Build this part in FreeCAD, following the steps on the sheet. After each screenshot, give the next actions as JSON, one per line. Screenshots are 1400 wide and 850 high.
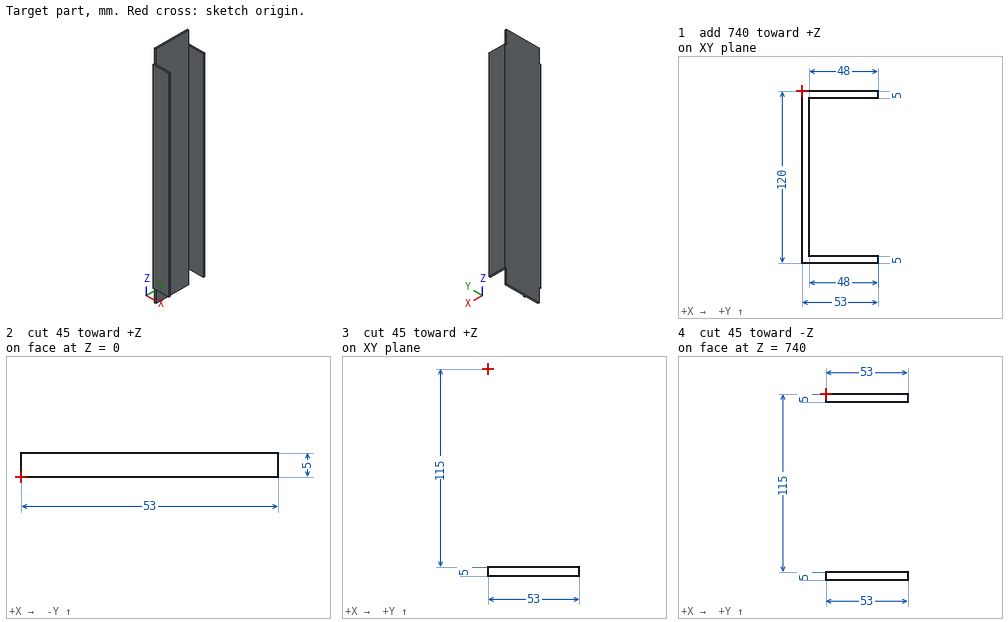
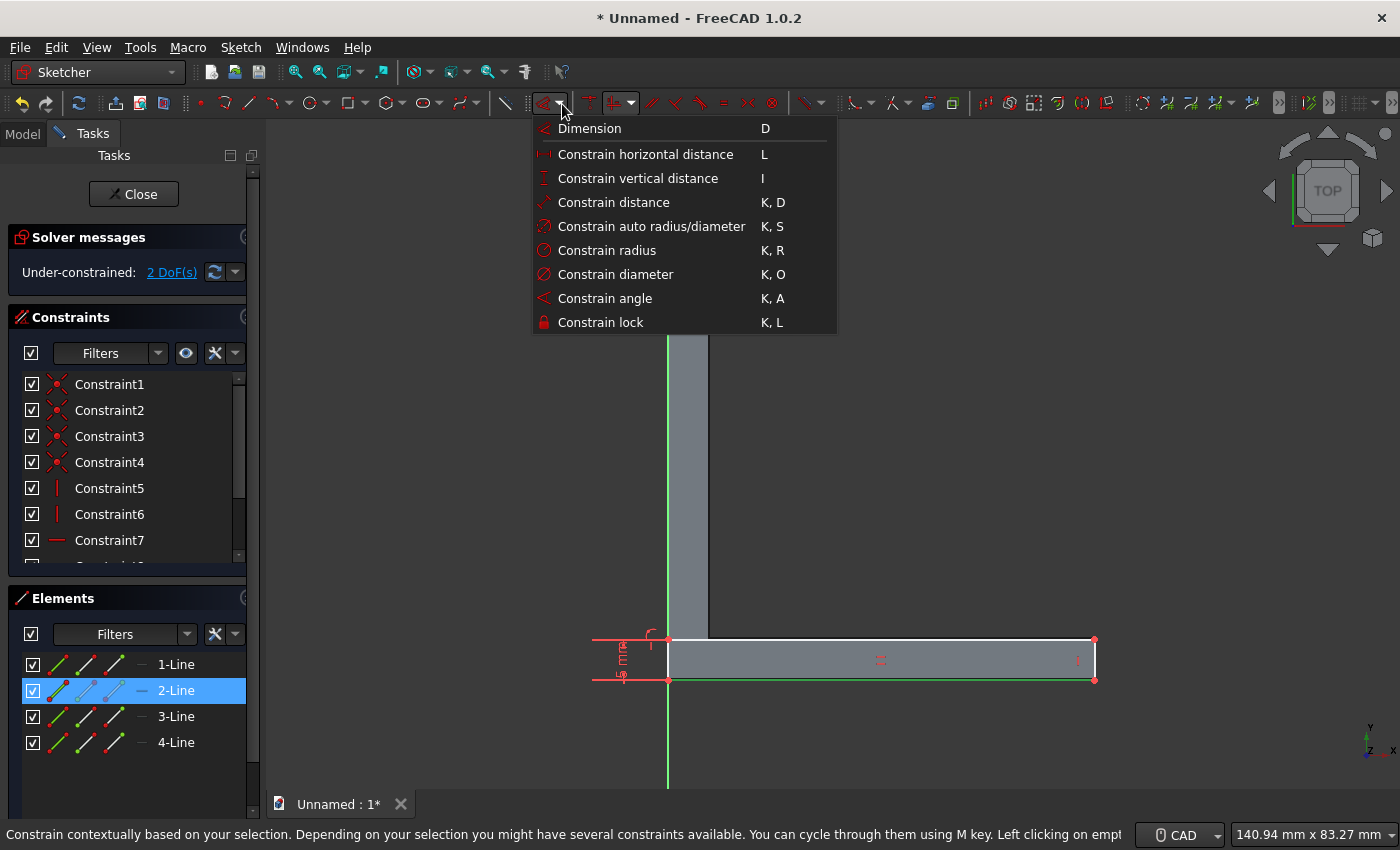
{"action": "left_click", "coordinate": [685, 154]}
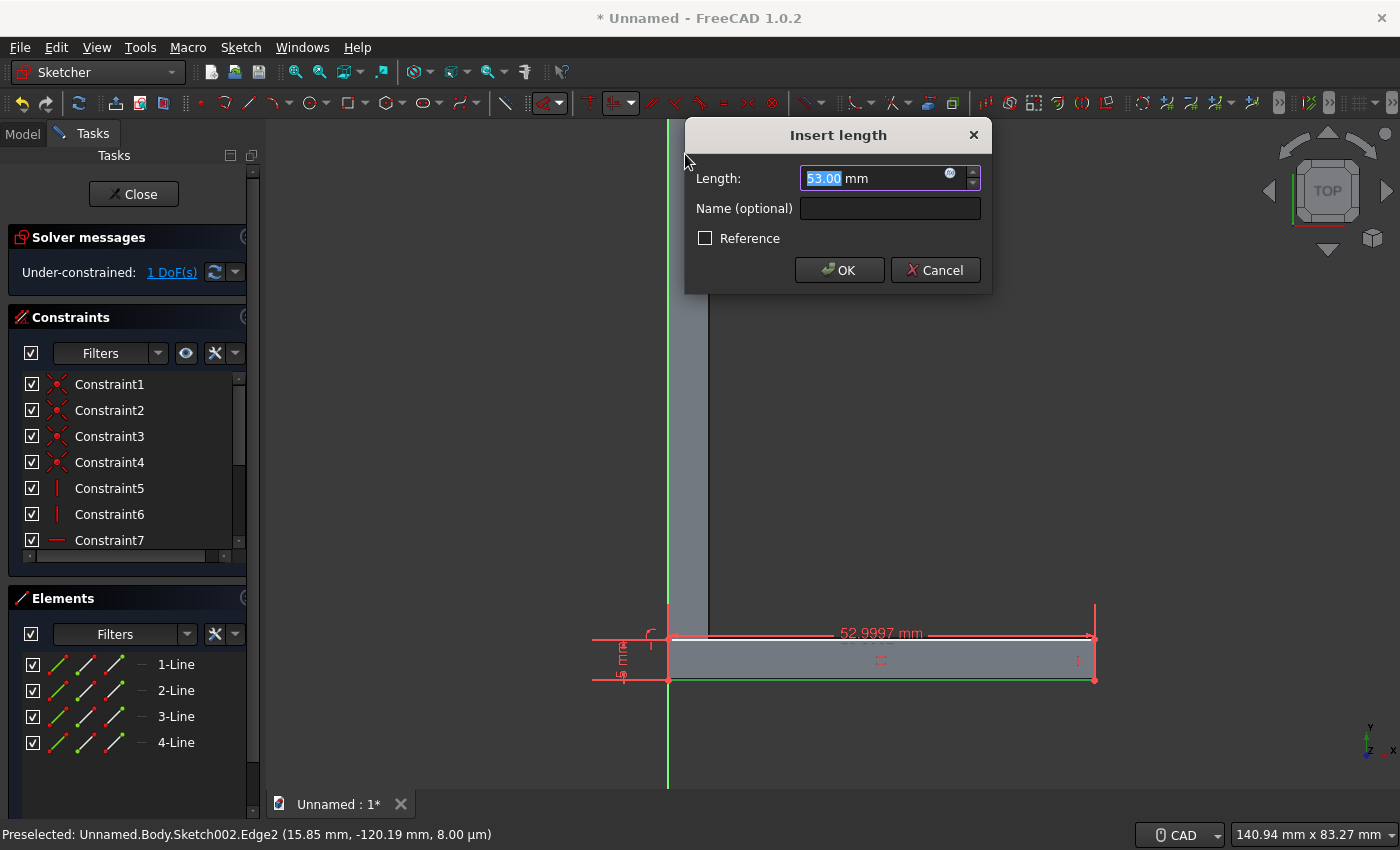
{"action": "type", "text": "53"}
{"action": "key", "text": "Return"}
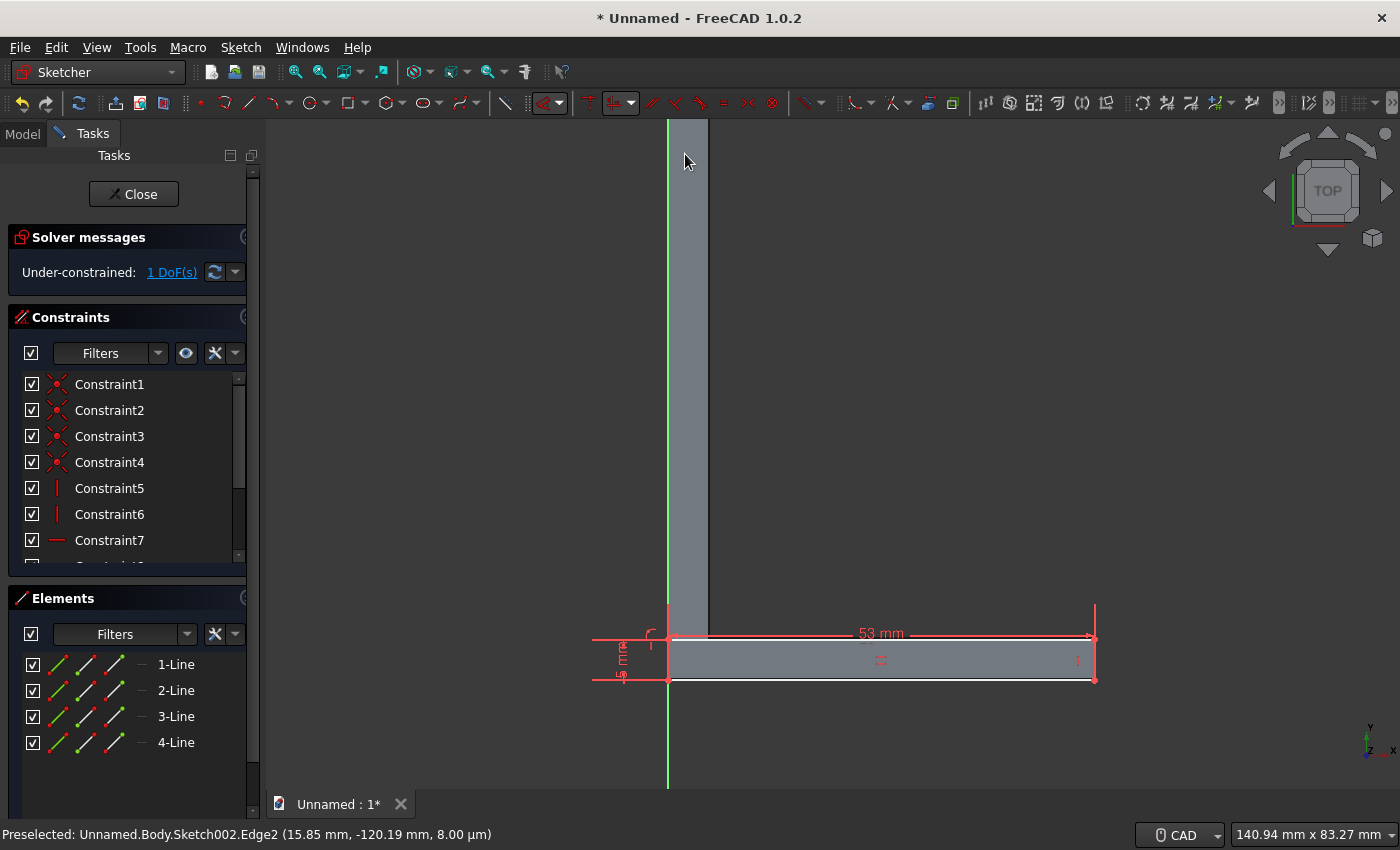
{"action": "left_click", "coordinate": [668, 640]}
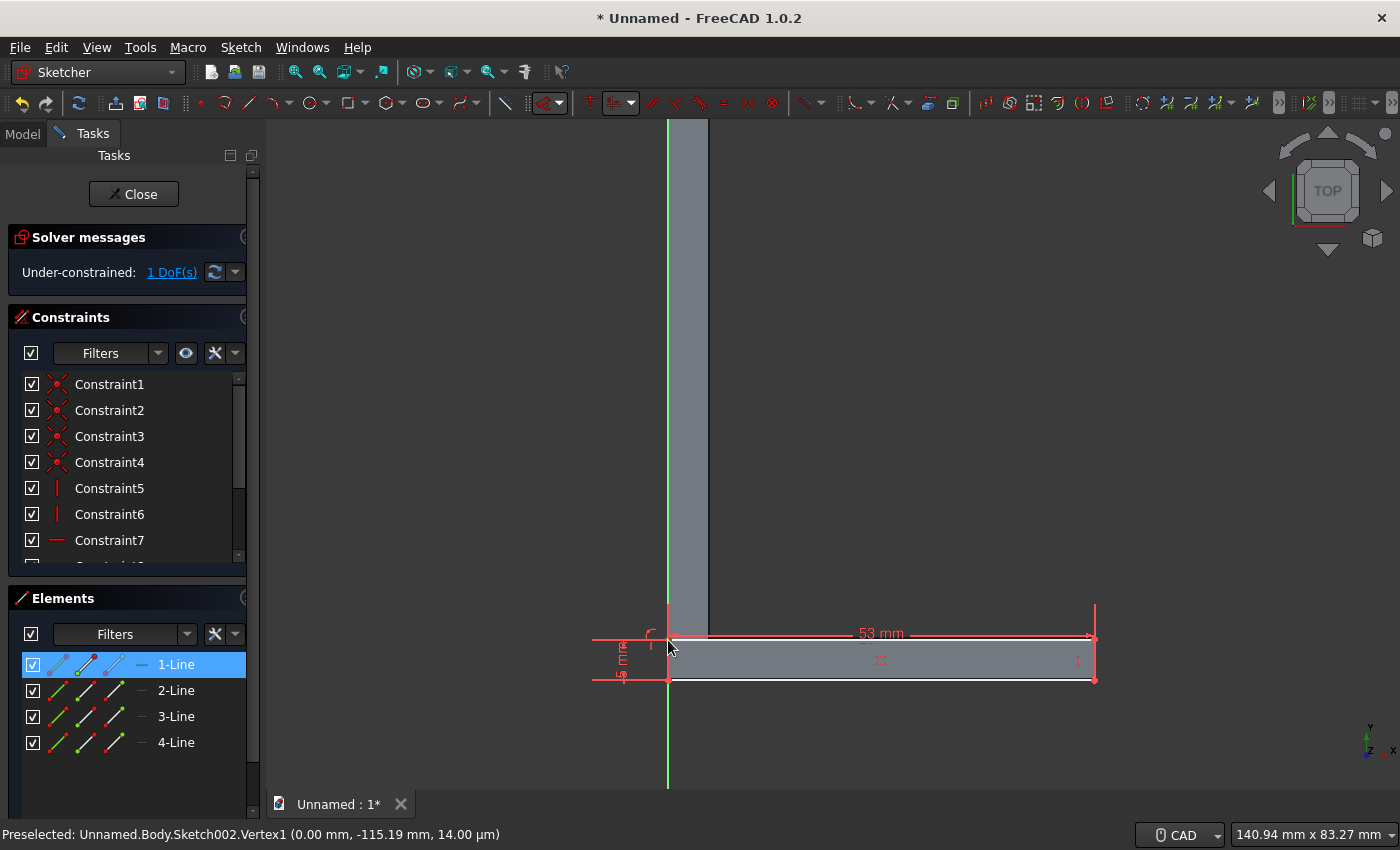
{"action": "key", "text": "i"}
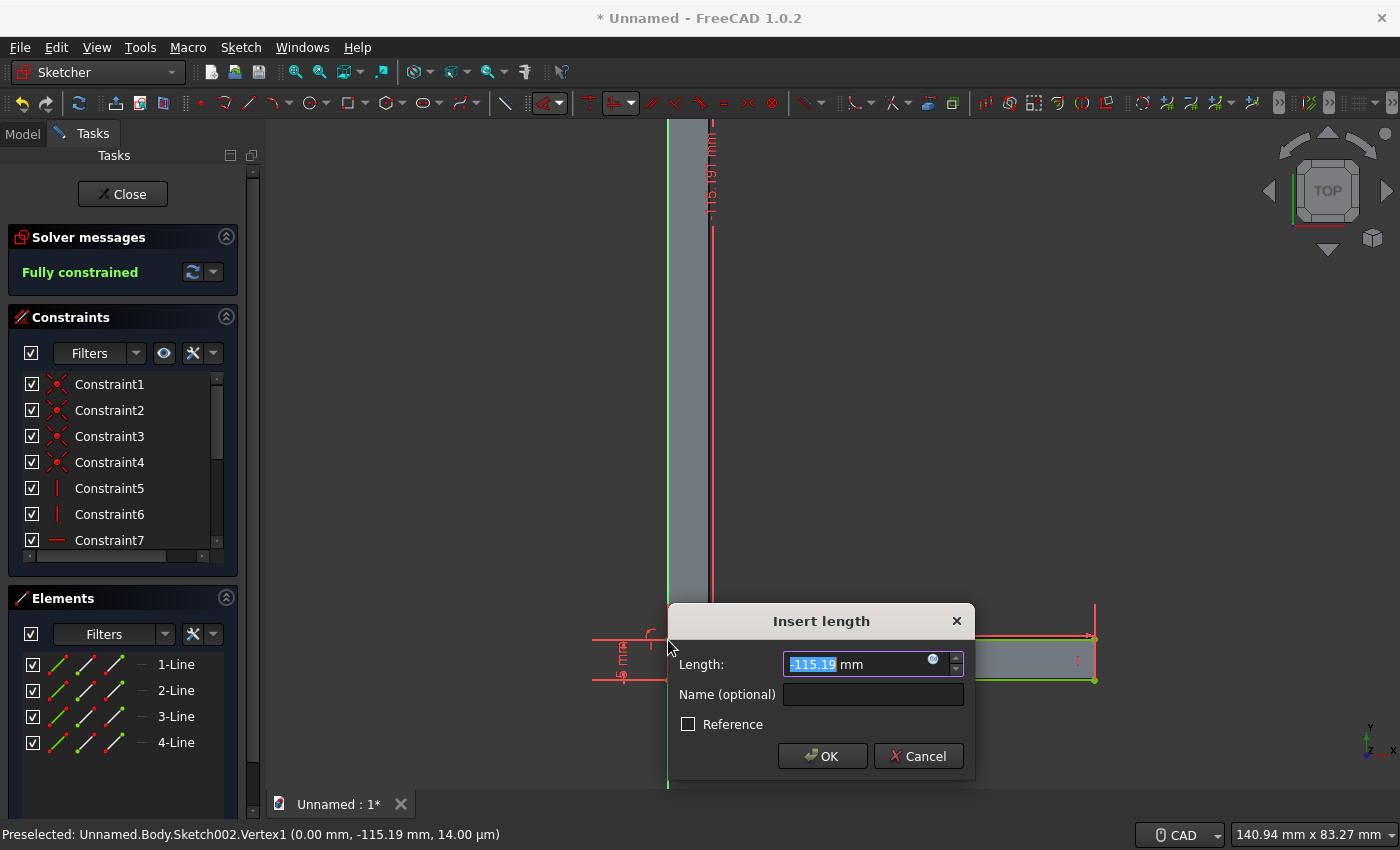
{"action": "type", "text": "-115"}
{"action": "key", "text": "Return"}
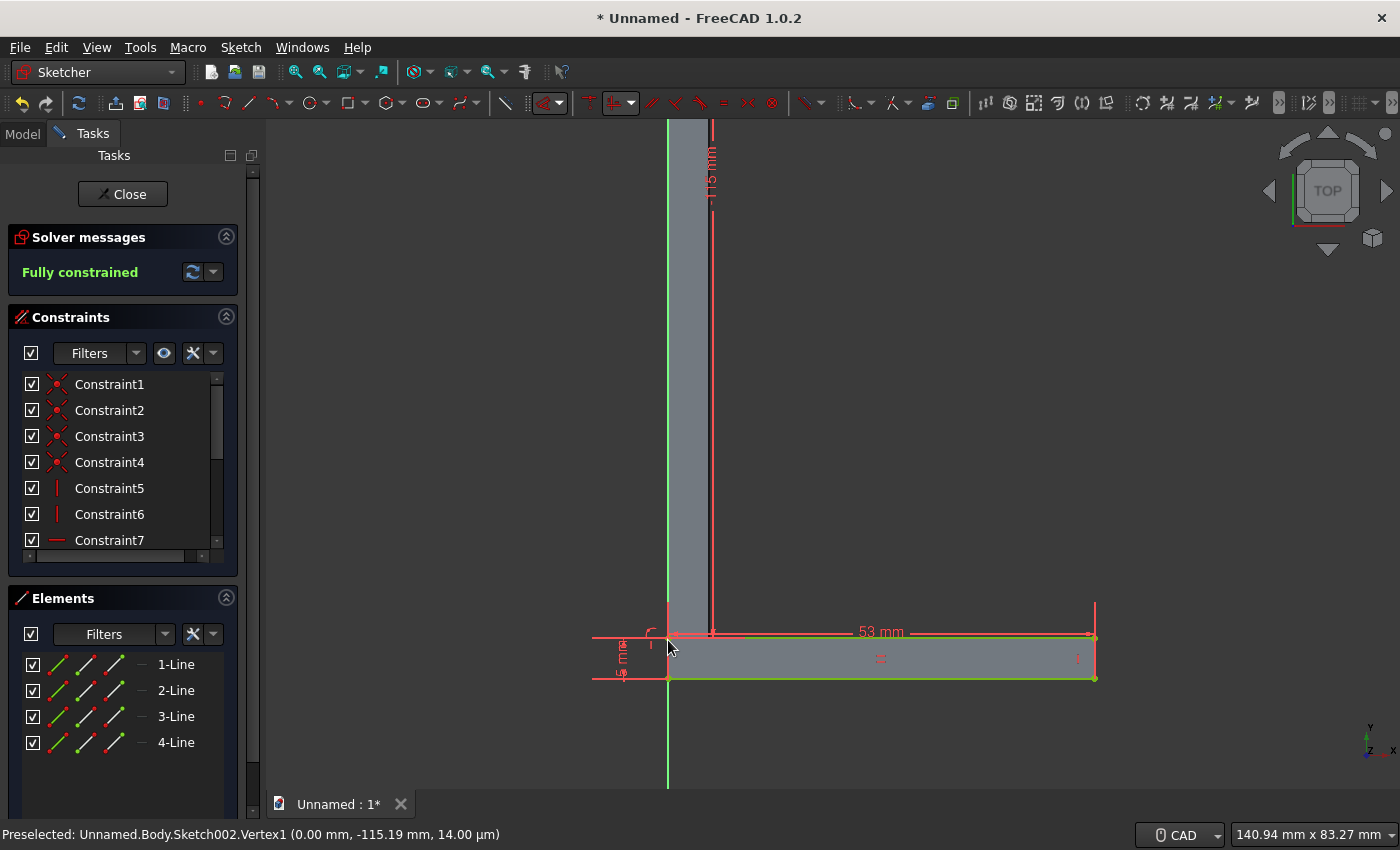
{"action": "left_click", "coordinate": [123, 194]}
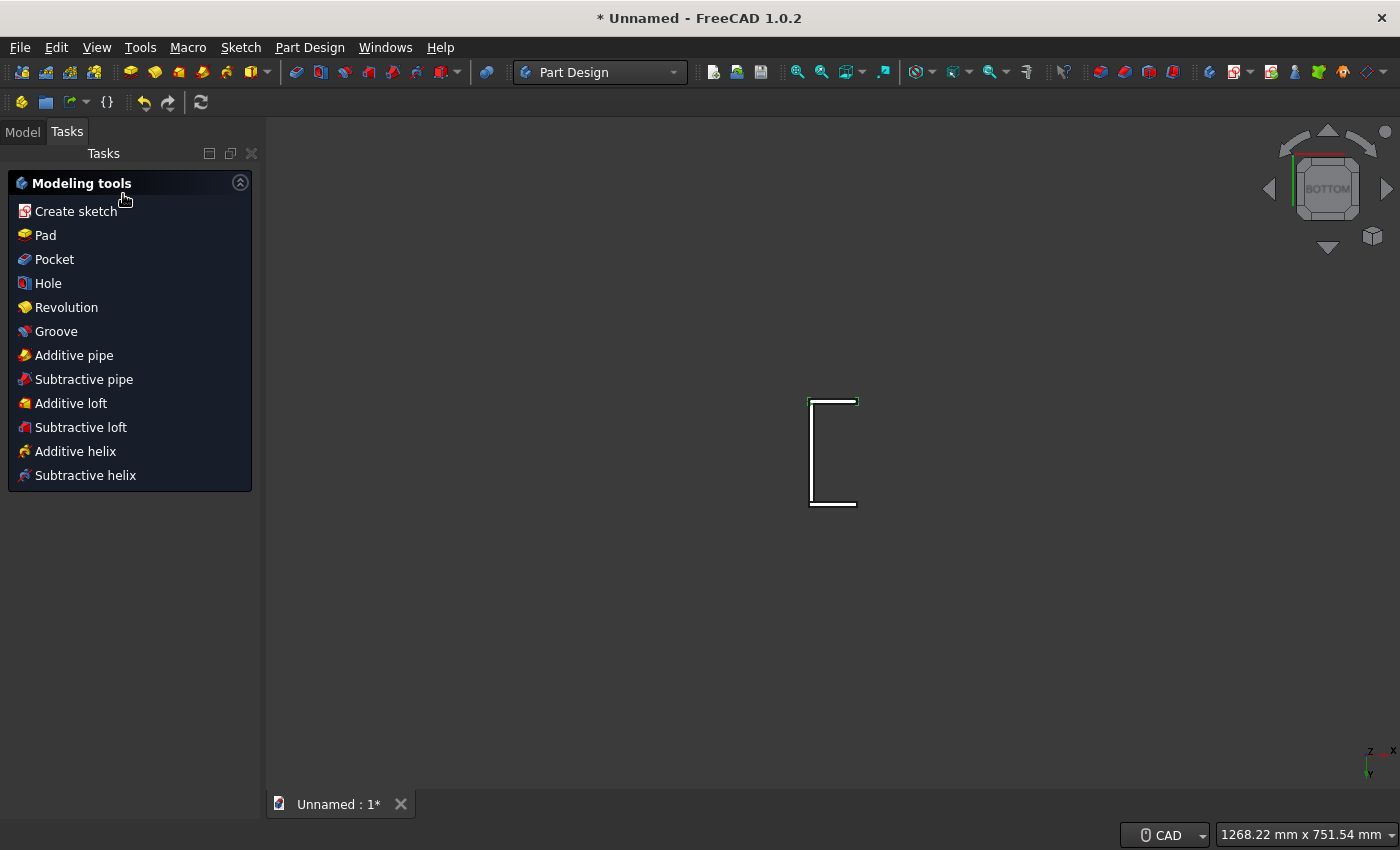
{"action": "left_click", "coordinate": [298, 72]}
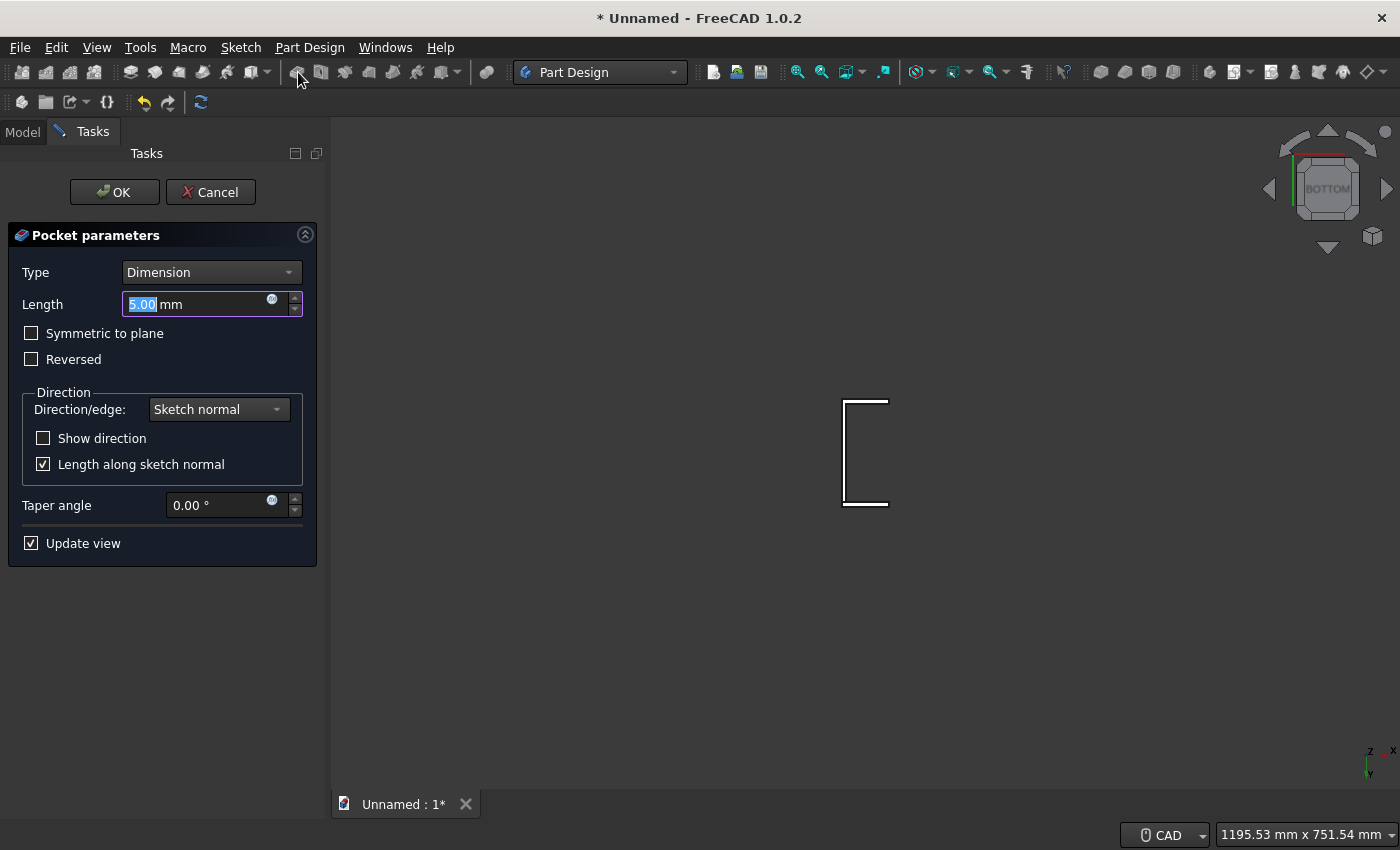
{"action": "type", "text": "45"}
{"action": "key", "text": "Tab"}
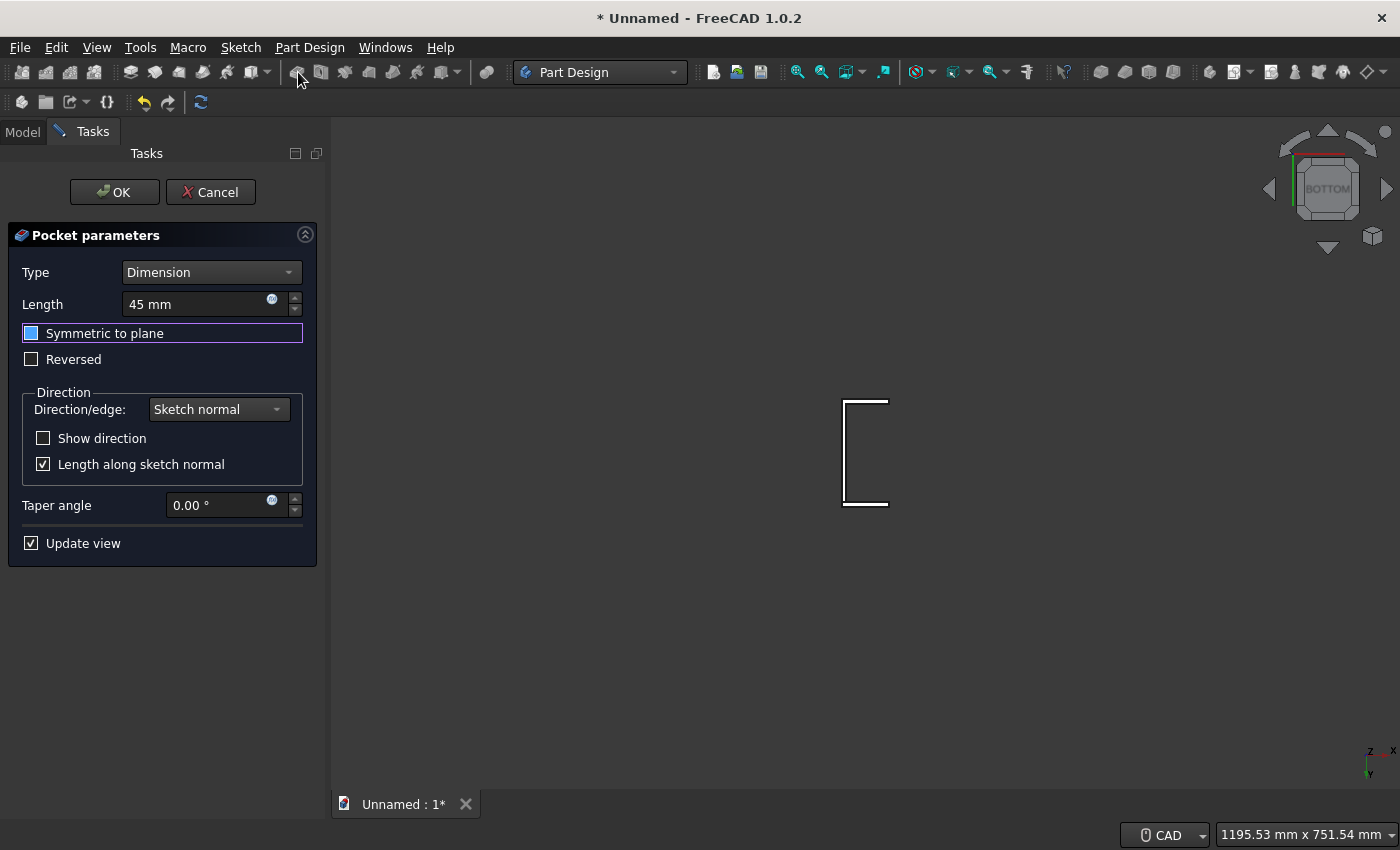
{"action": "left_click", "coordinate": [30, 359]}